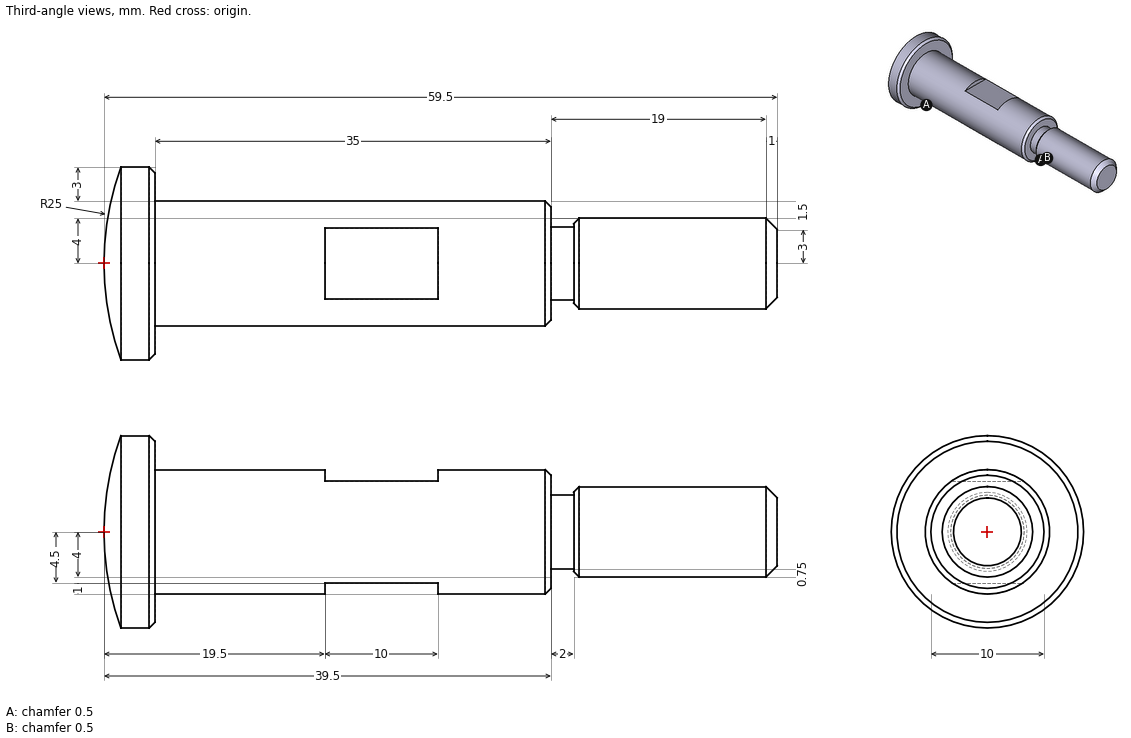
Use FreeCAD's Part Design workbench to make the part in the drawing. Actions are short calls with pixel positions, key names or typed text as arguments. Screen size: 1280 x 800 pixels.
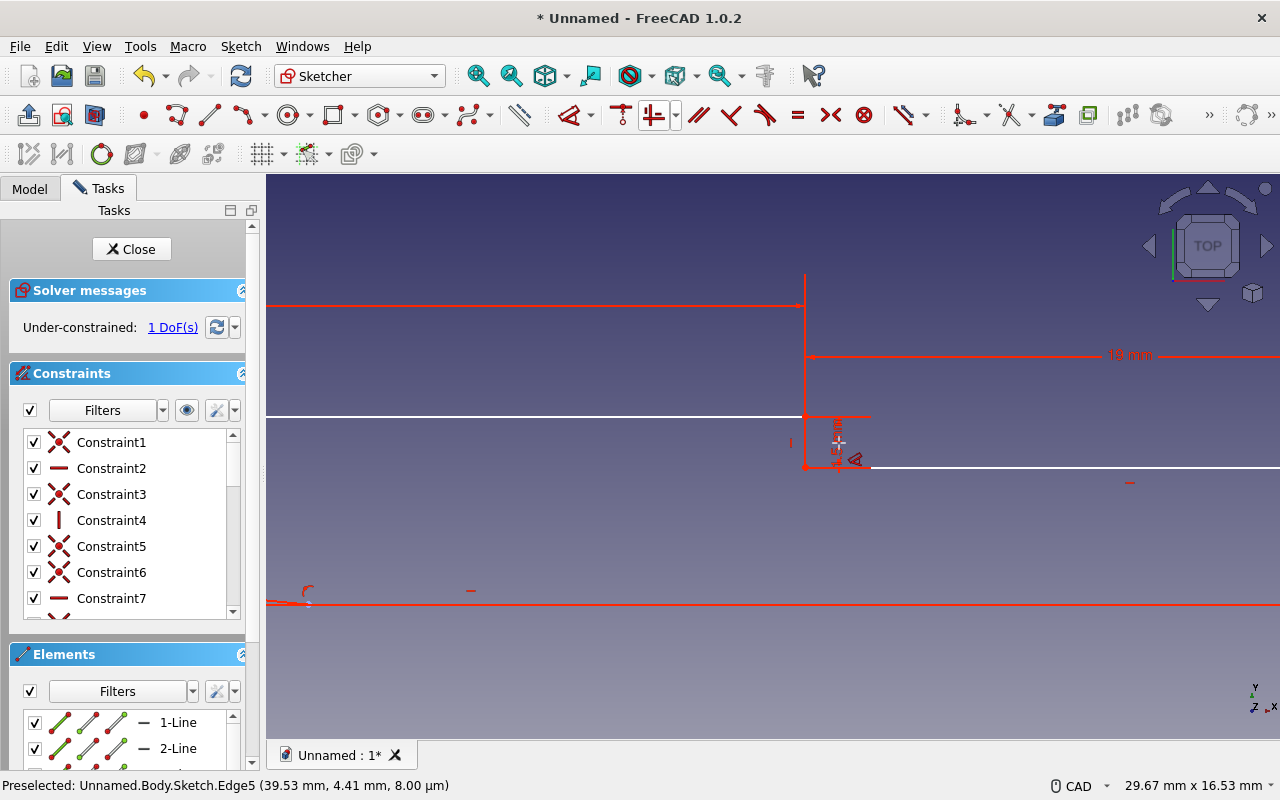
click(879, 605)
click(704, 639)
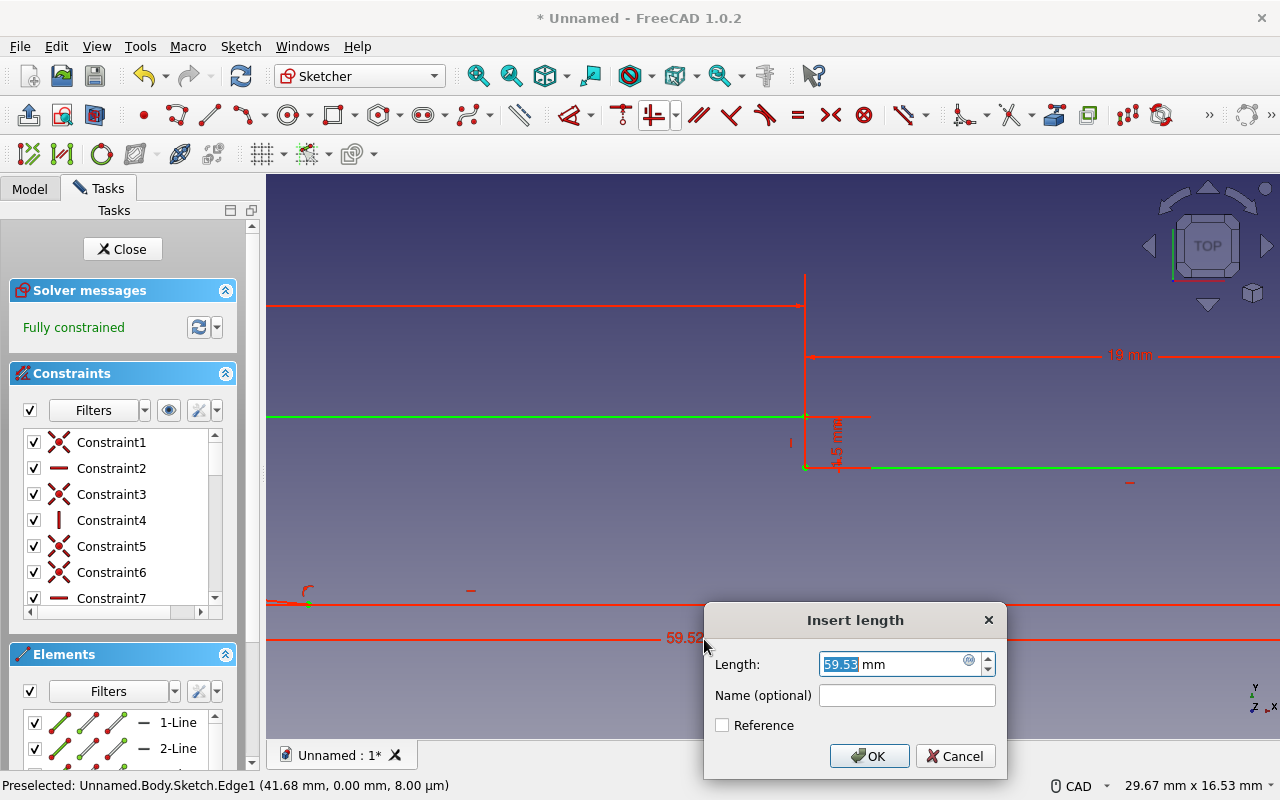
text(59.5)
key(Return)
key(Escape)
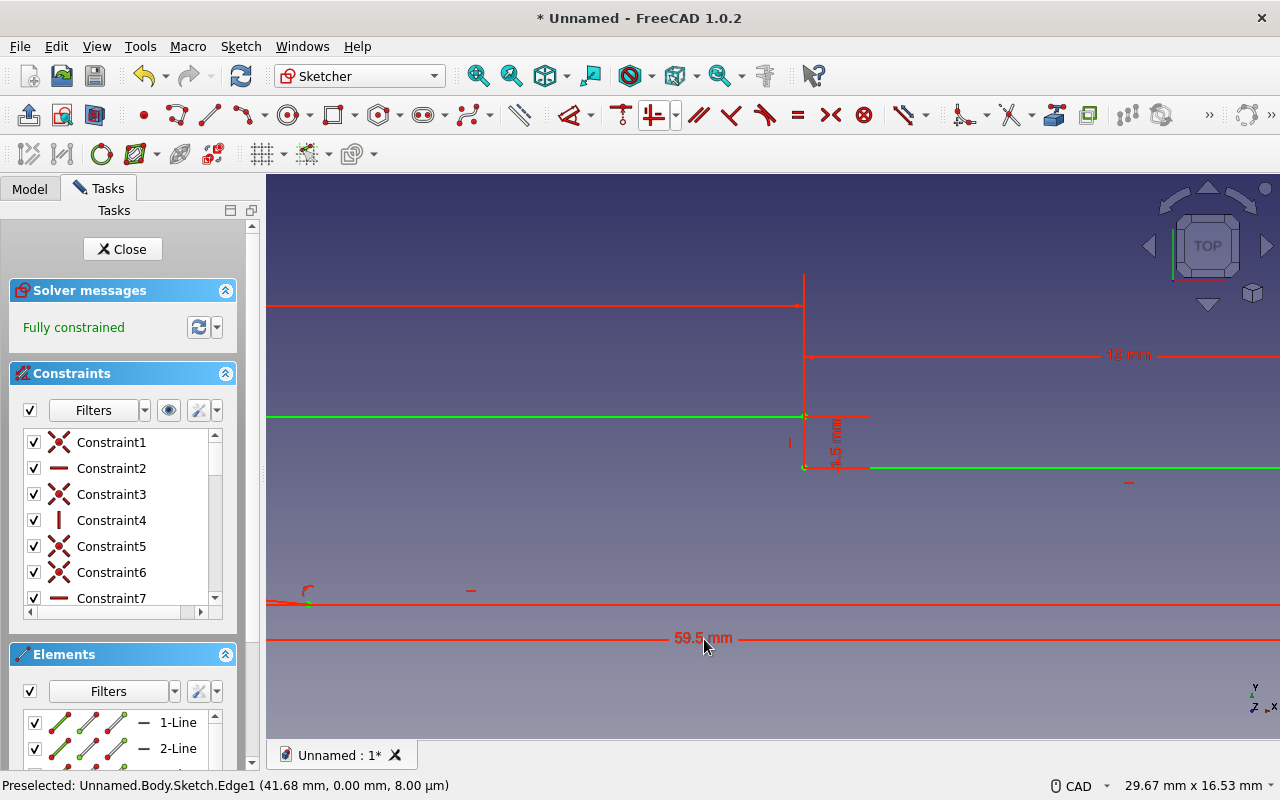
click(123, 249)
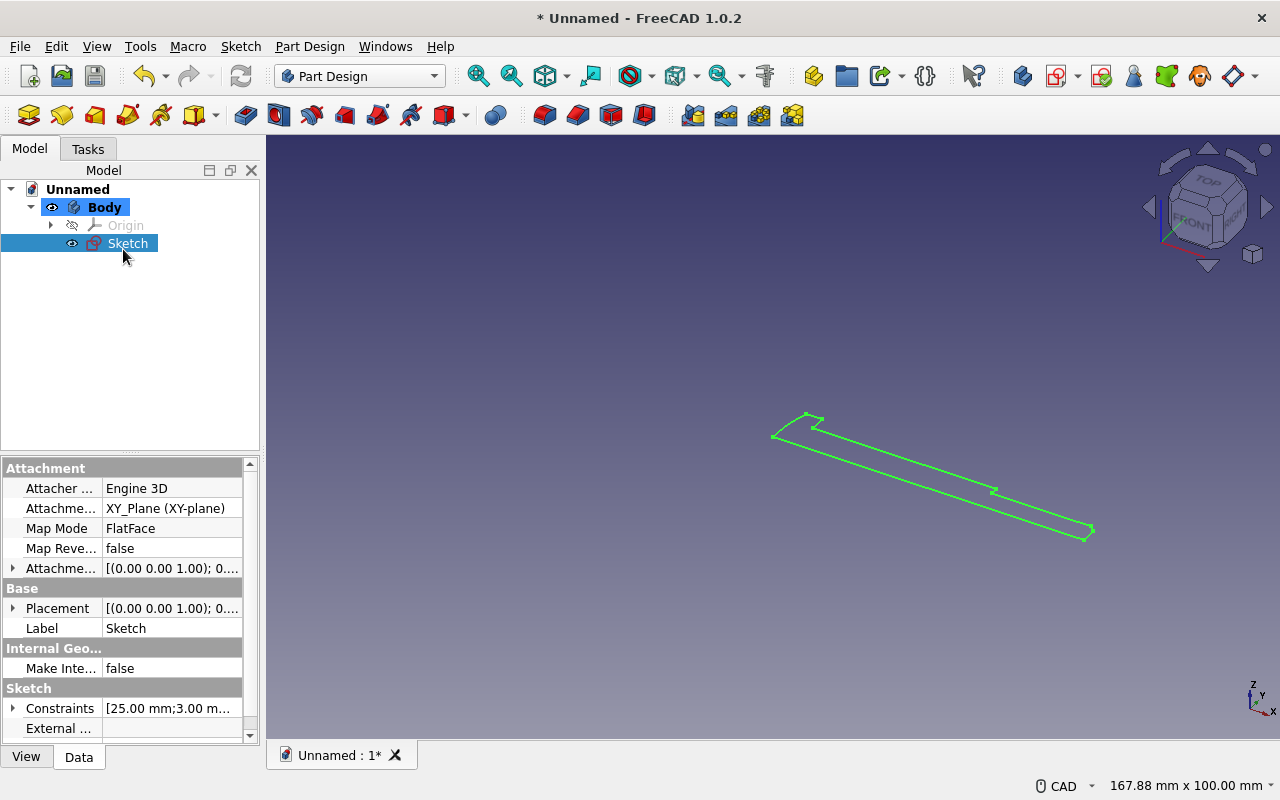
click(62, 116)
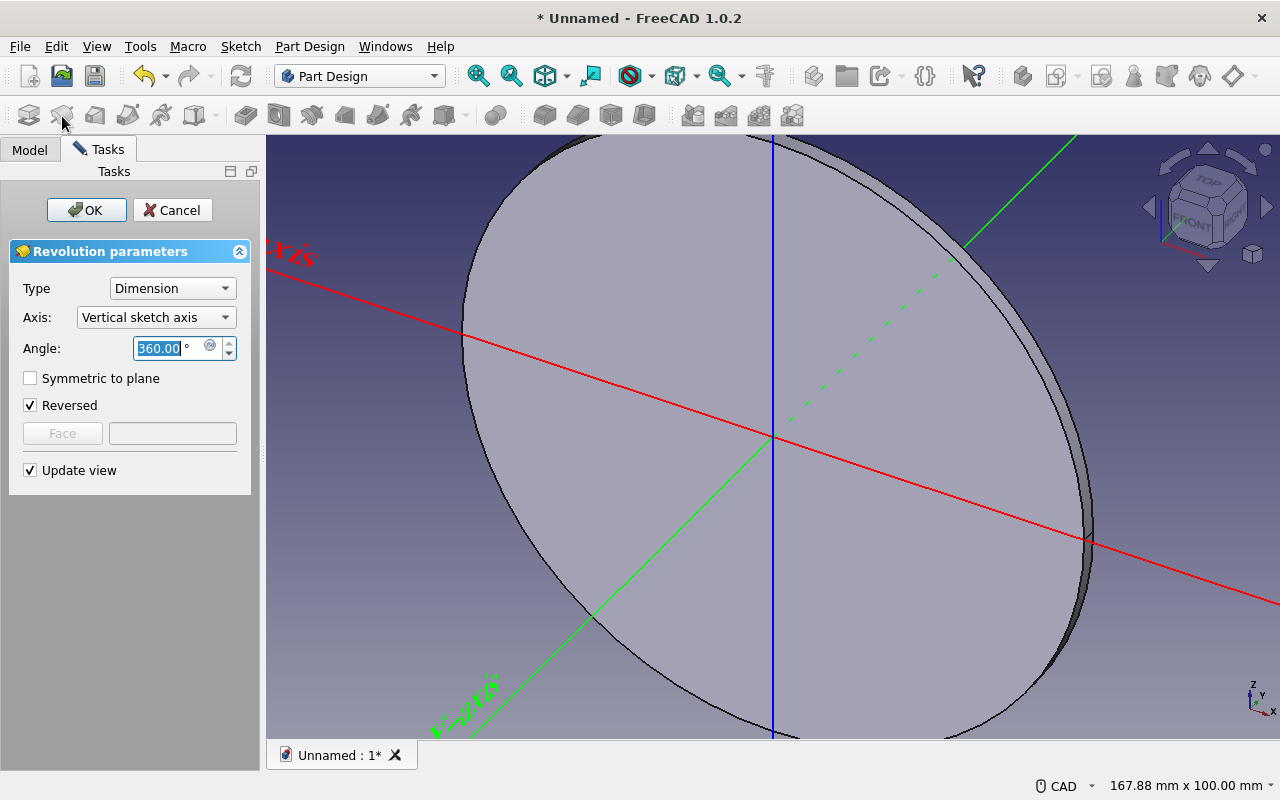
click(157, 318)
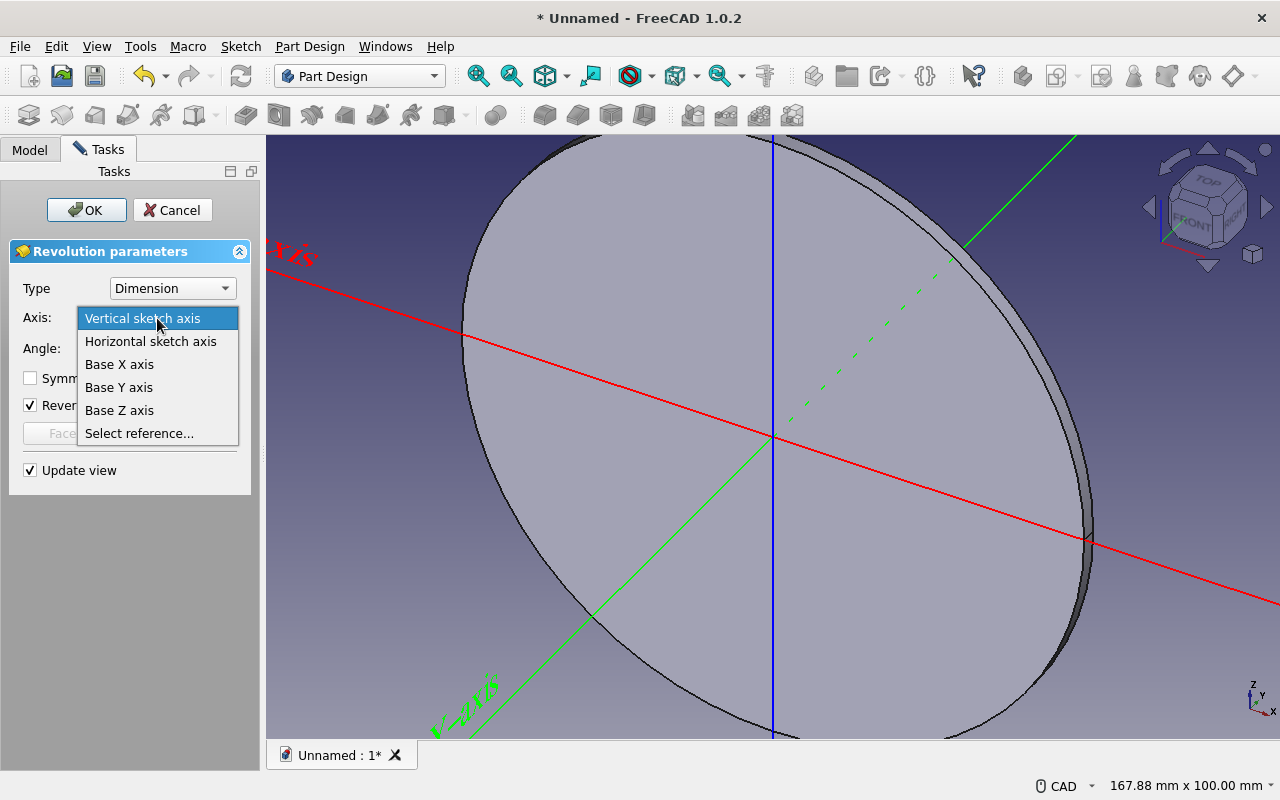
click(156, 342)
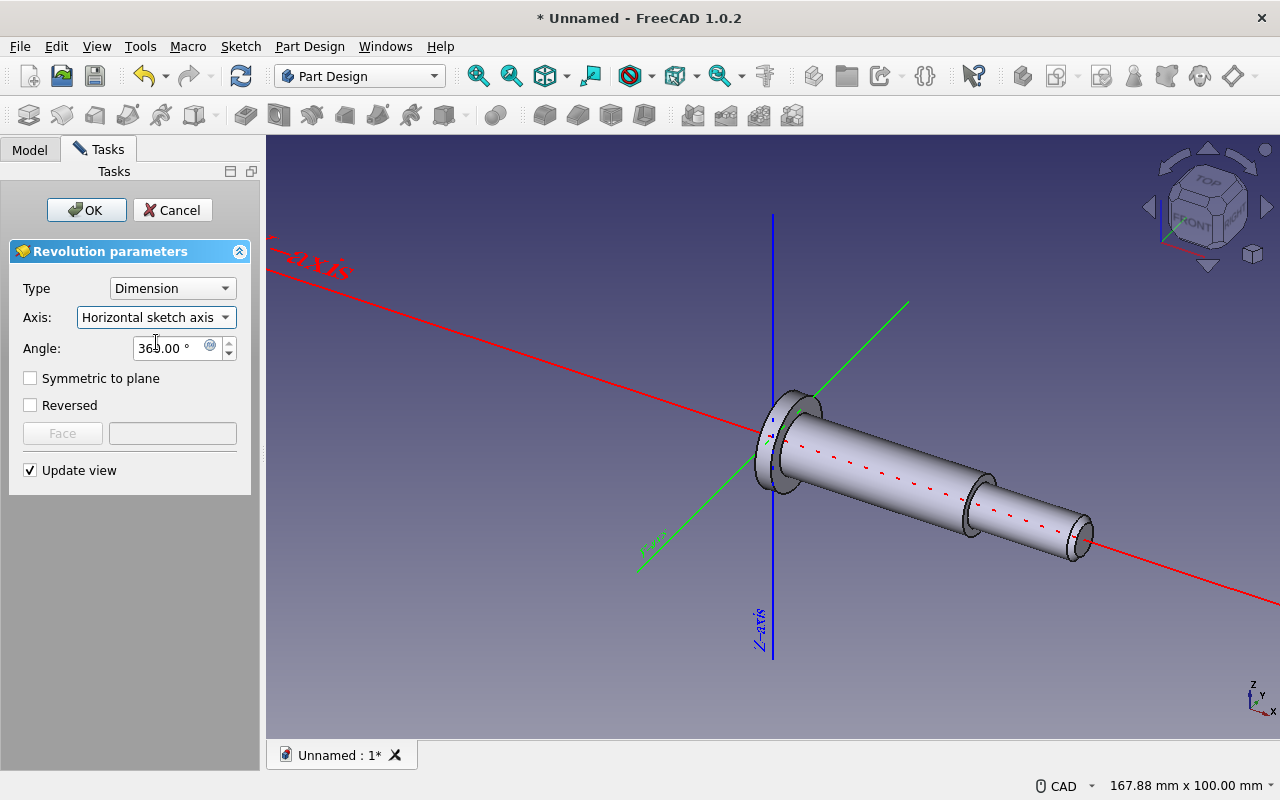
click(87, 210)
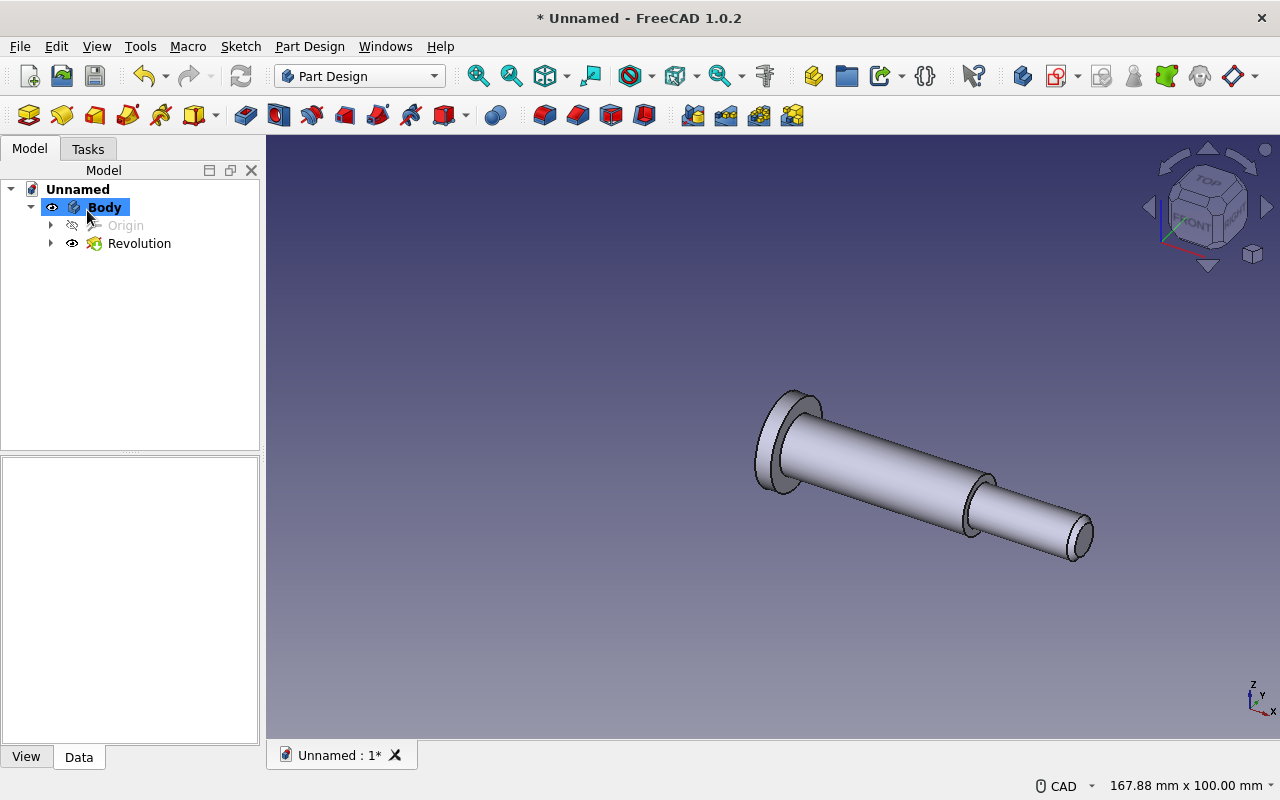
click(479, 76)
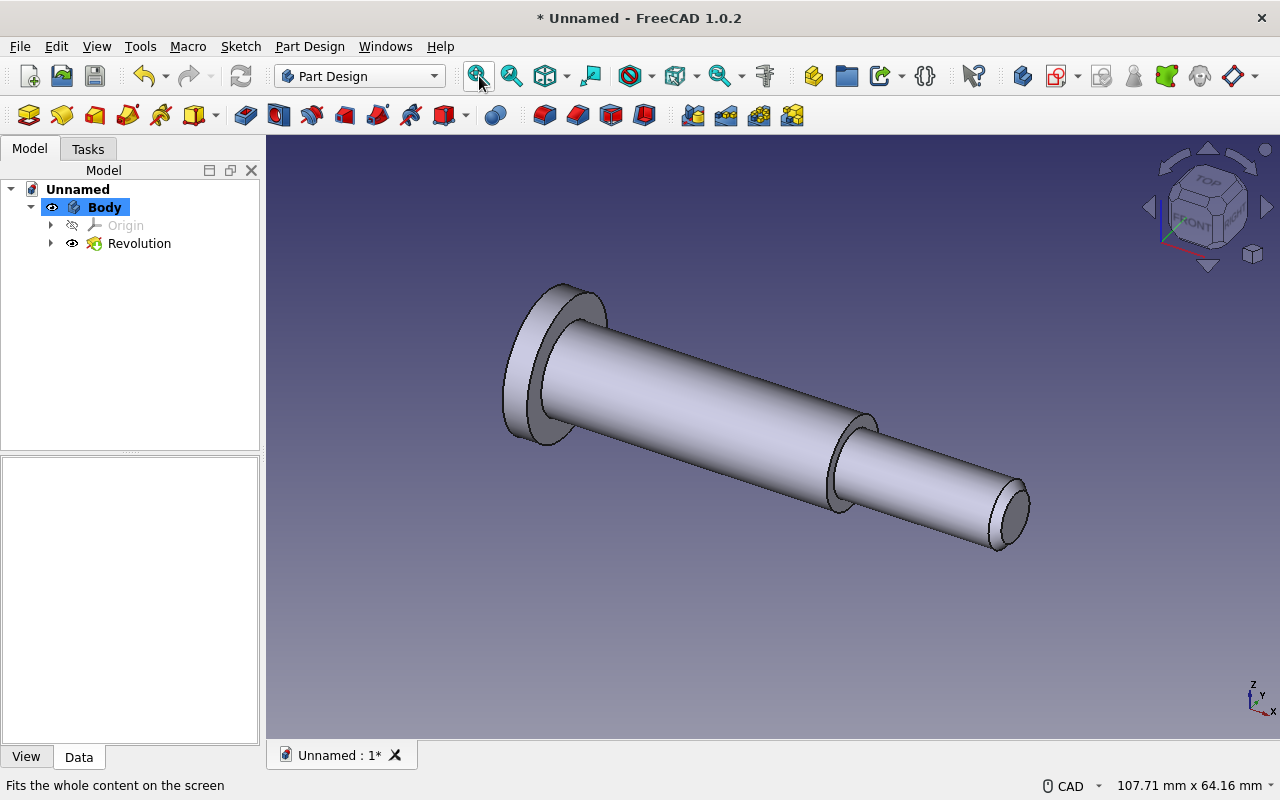
click(1056, 76)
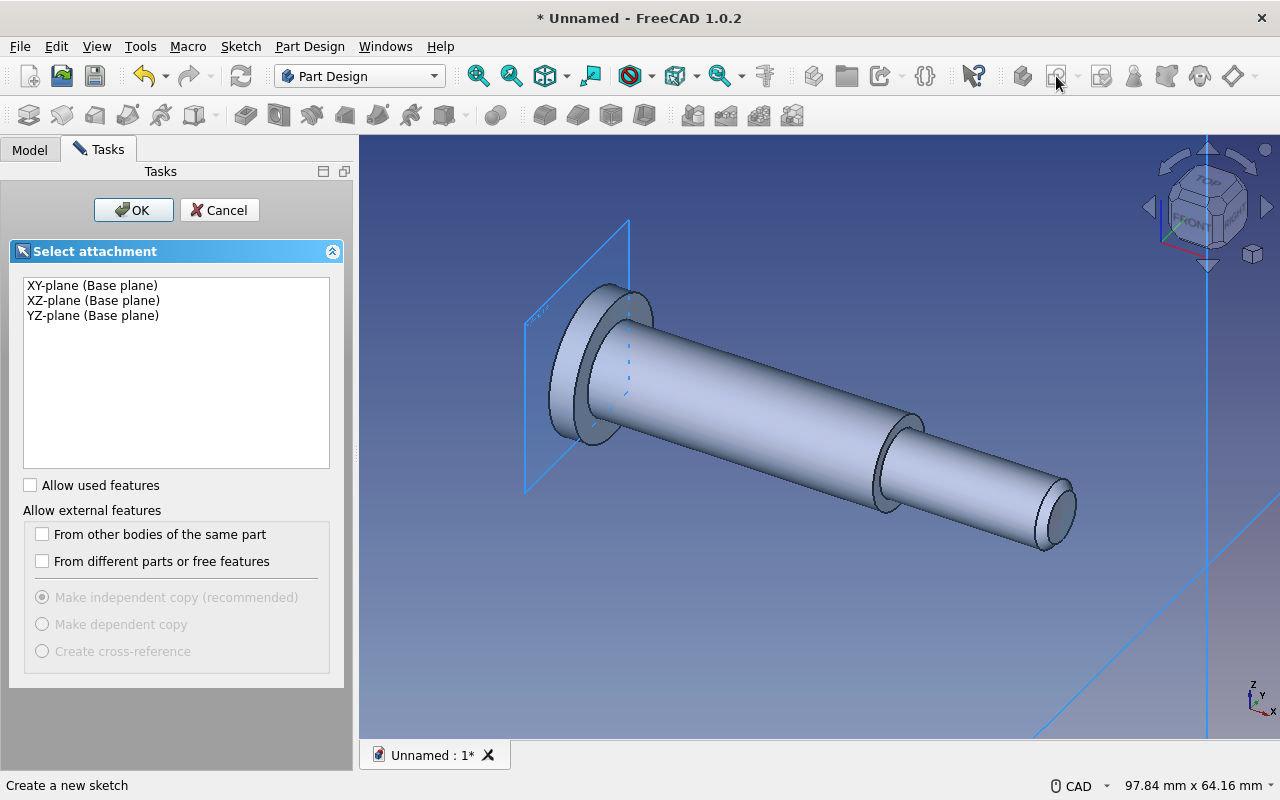
click(84, 300)